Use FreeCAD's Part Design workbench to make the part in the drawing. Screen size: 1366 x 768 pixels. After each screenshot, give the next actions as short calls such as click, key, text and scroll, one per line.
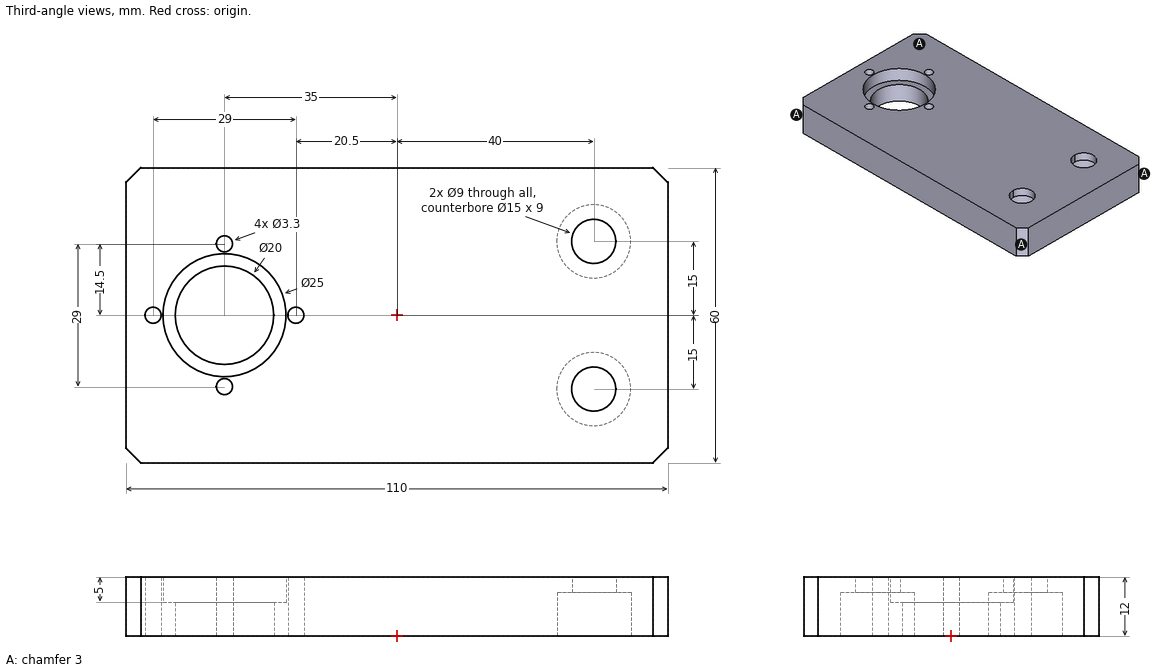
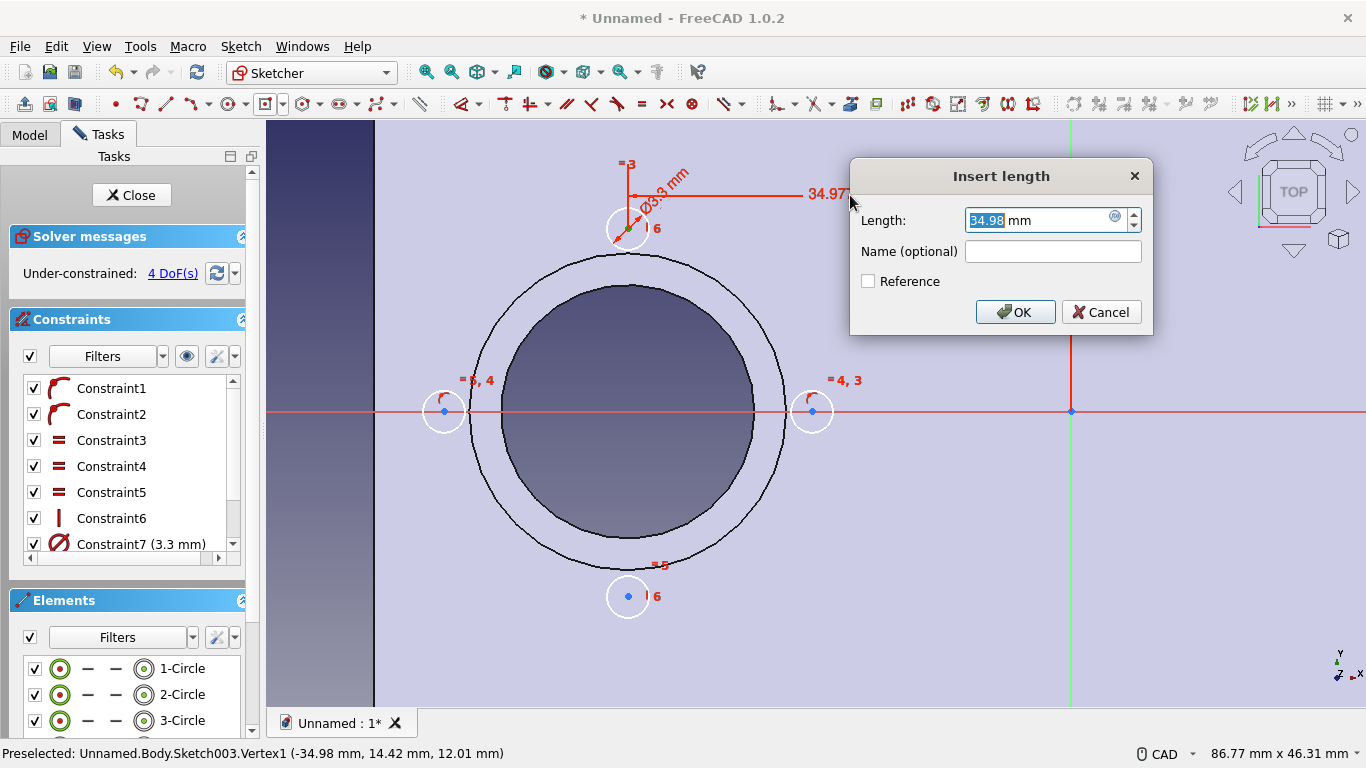
text(35)
key(Return)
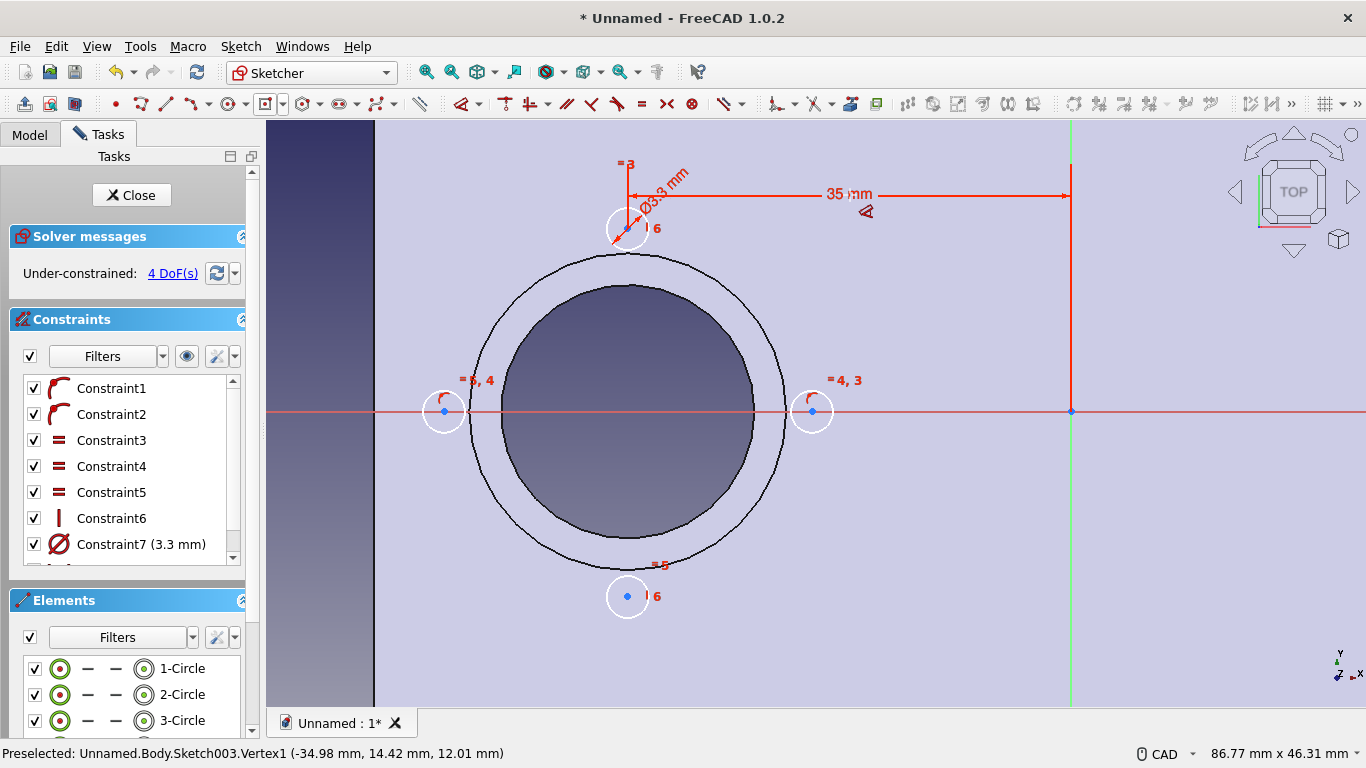
click(812, 412)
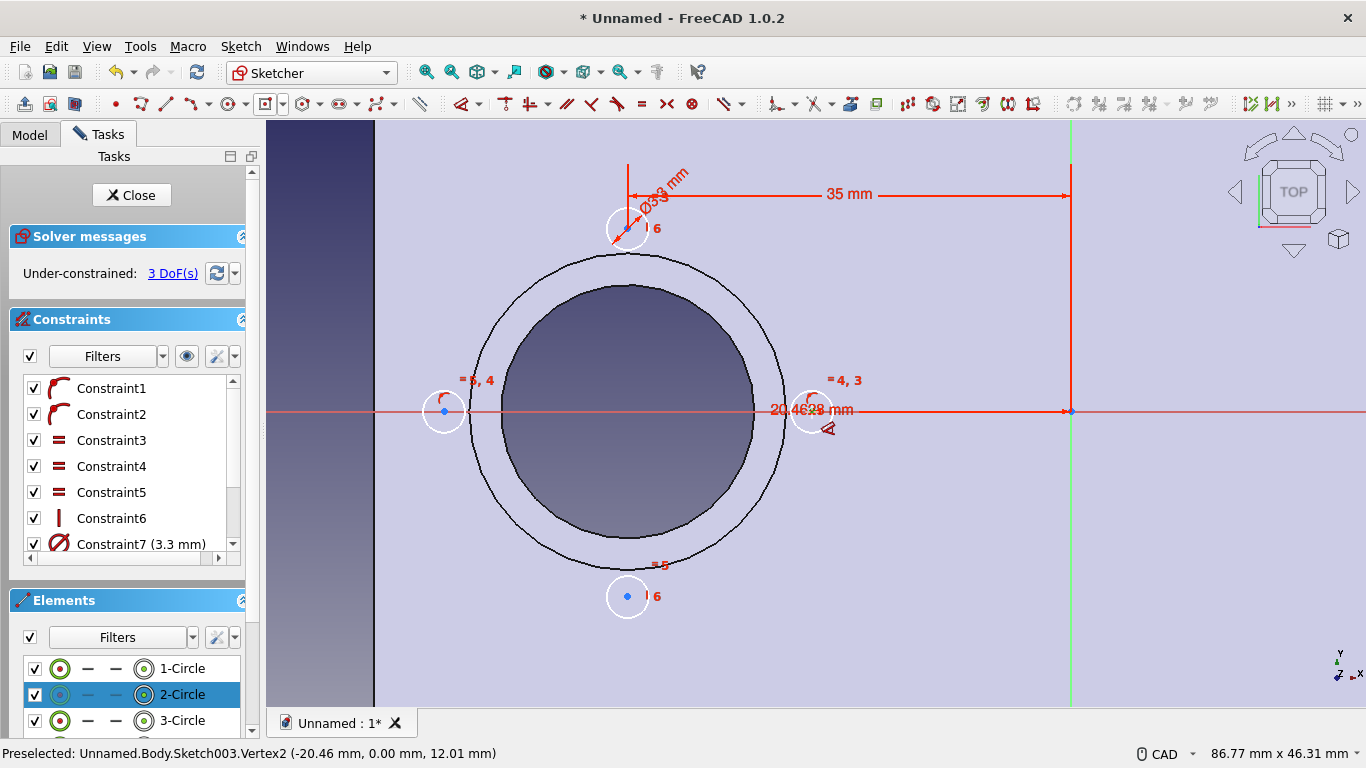
click(444, 412)
click(628, 446)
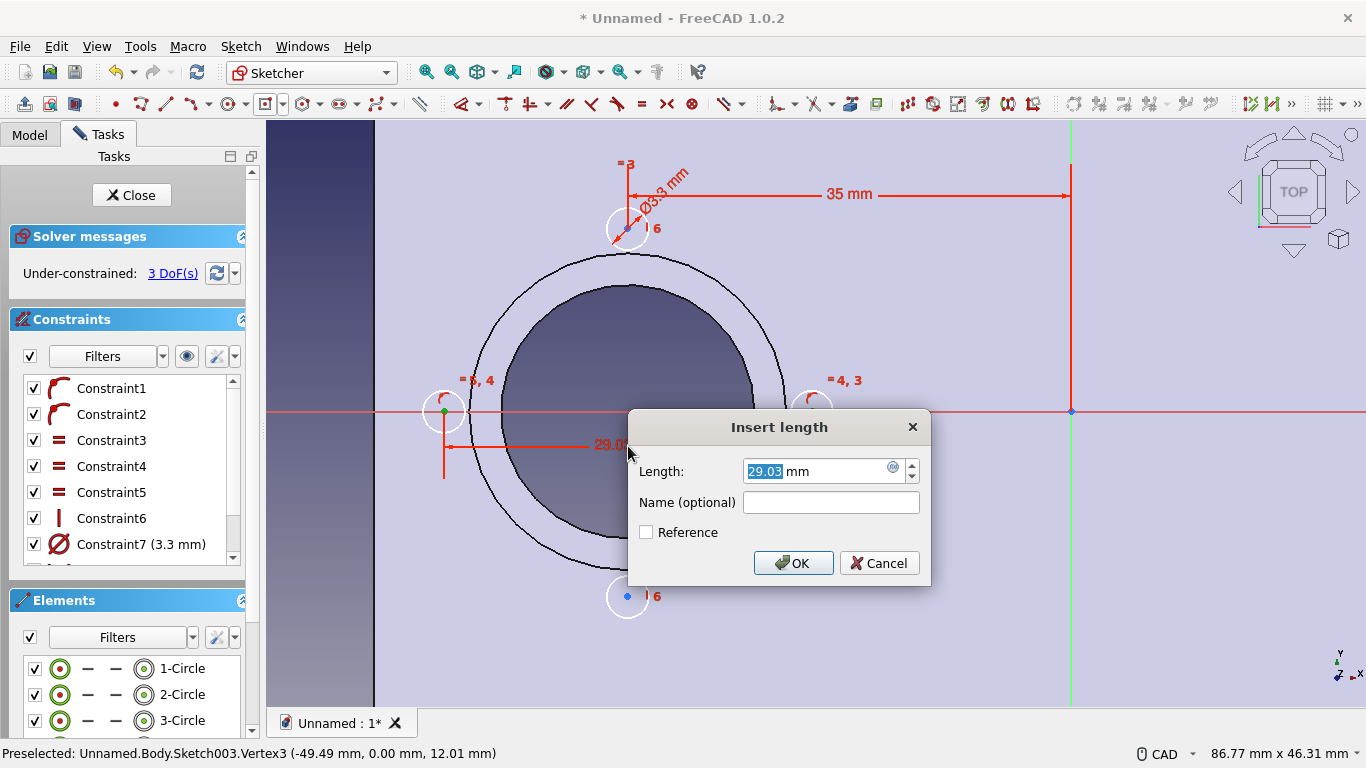
text(29)
key(Return)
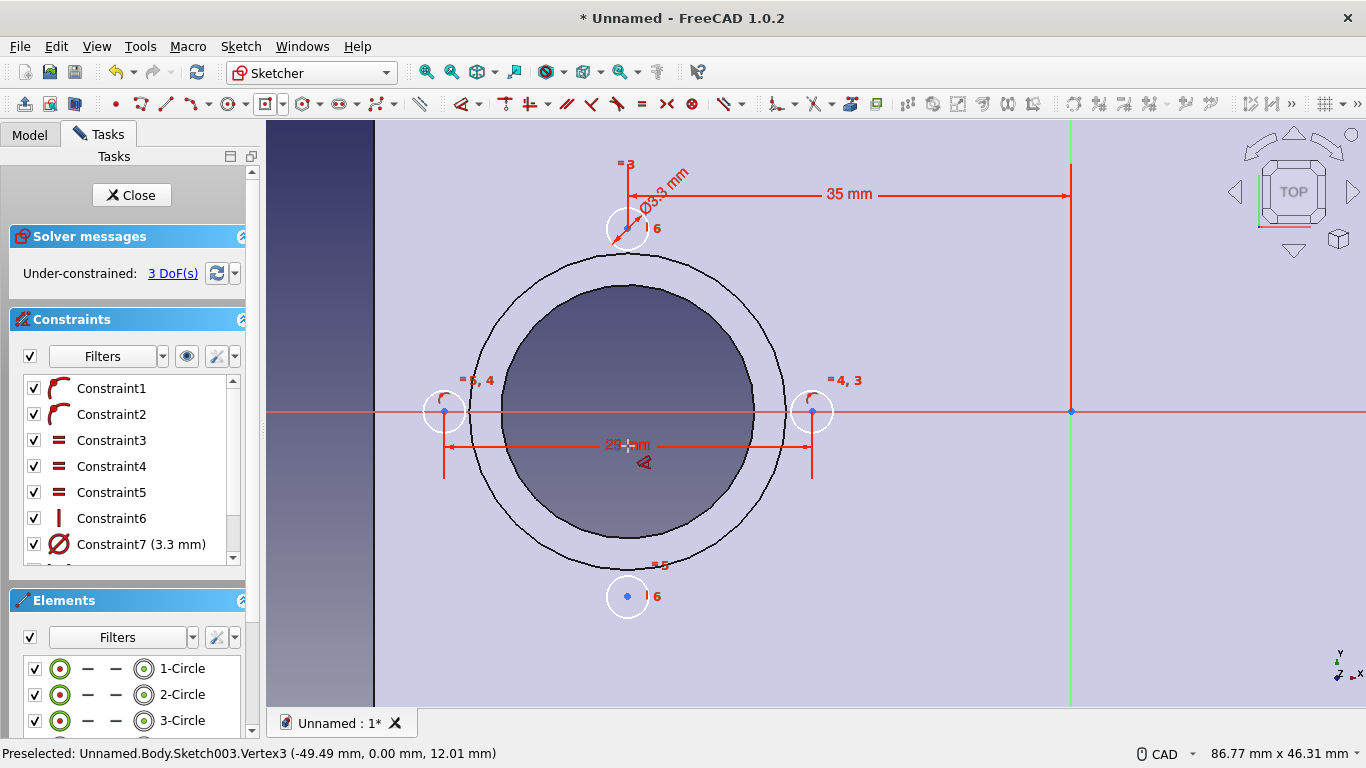
click(628, 229)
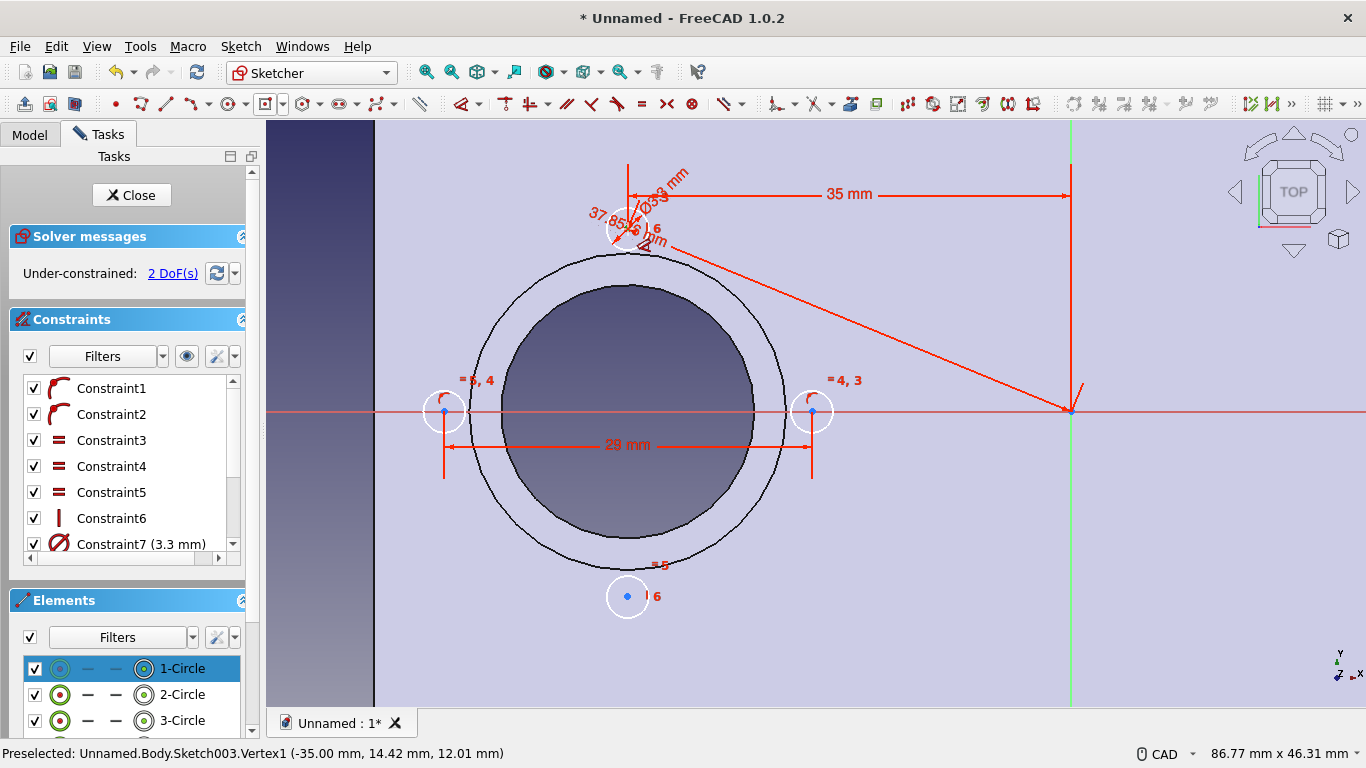
click(628, 597)
click(594, 328)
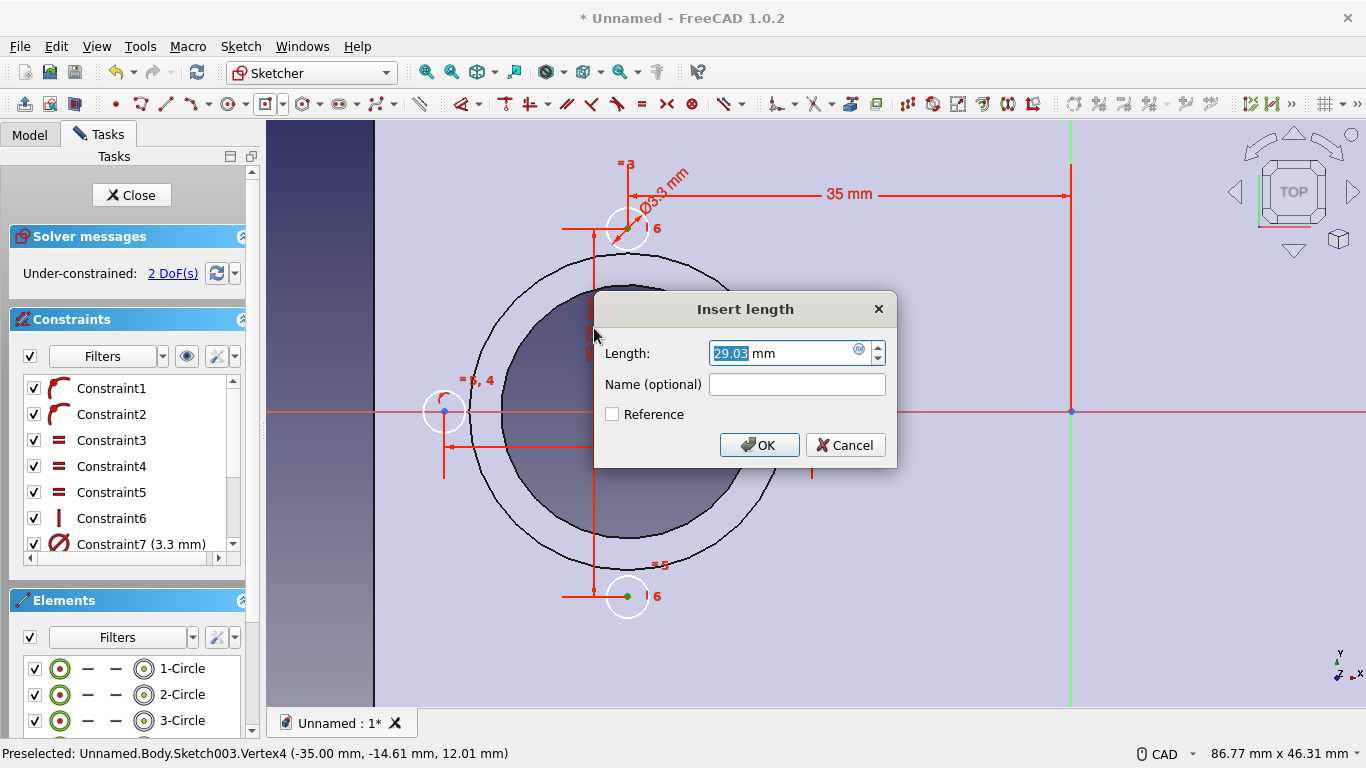
text(29)
key(Return)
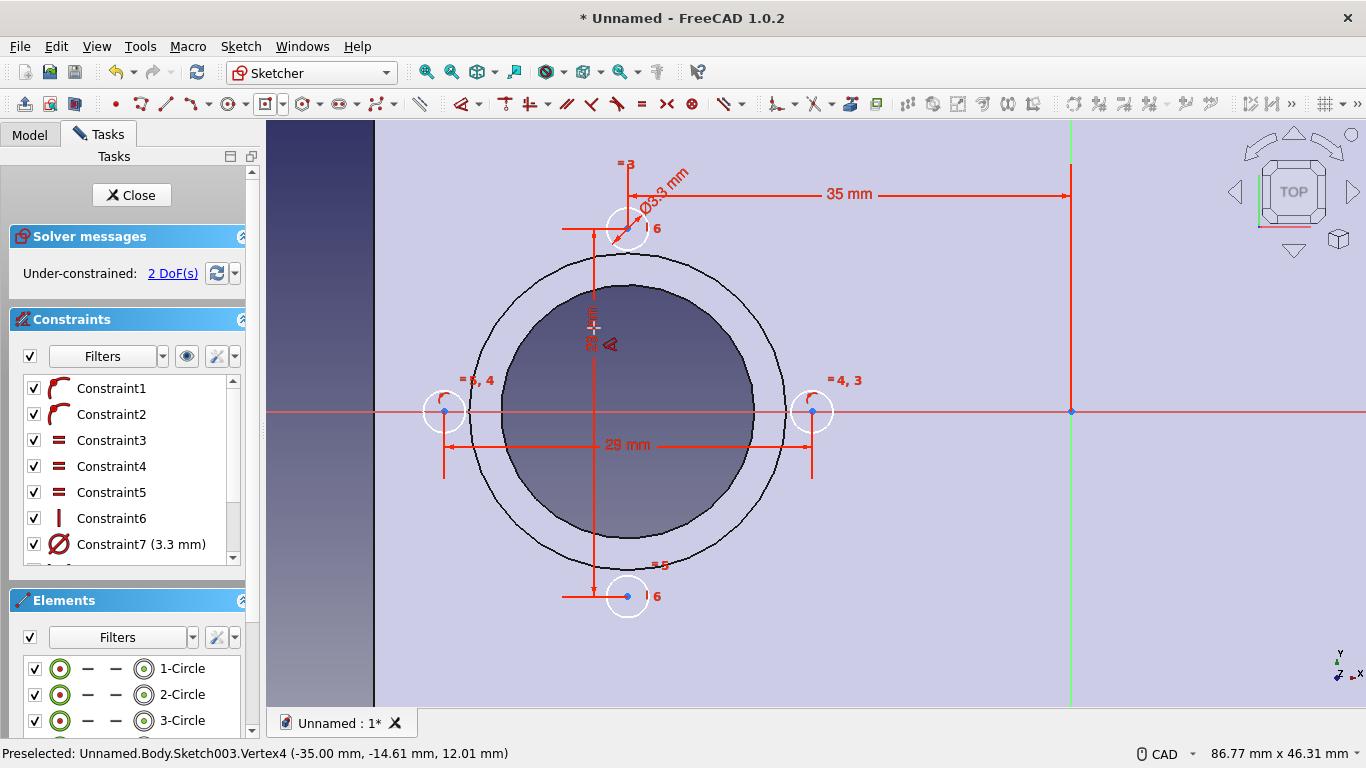
click(628, 229)
click(1105, 320)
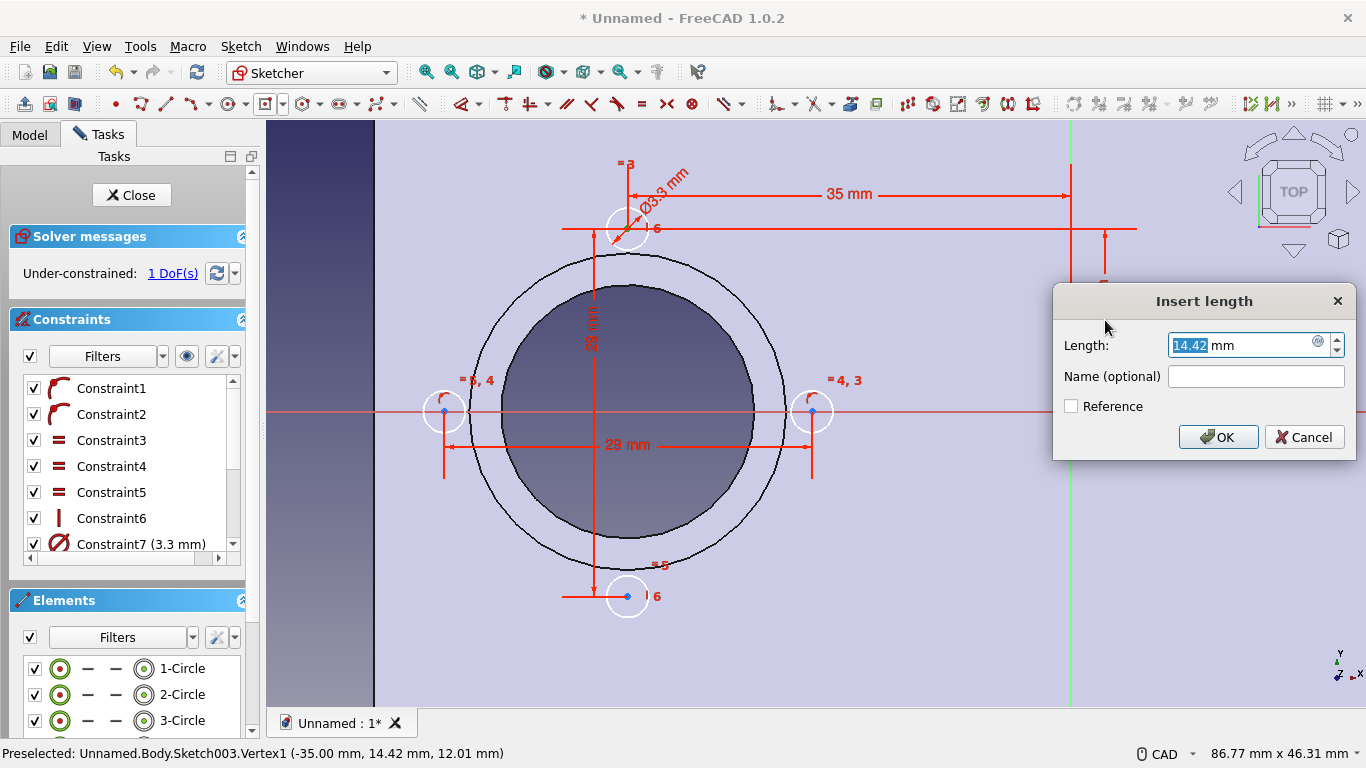
text(14.5)
key(Return)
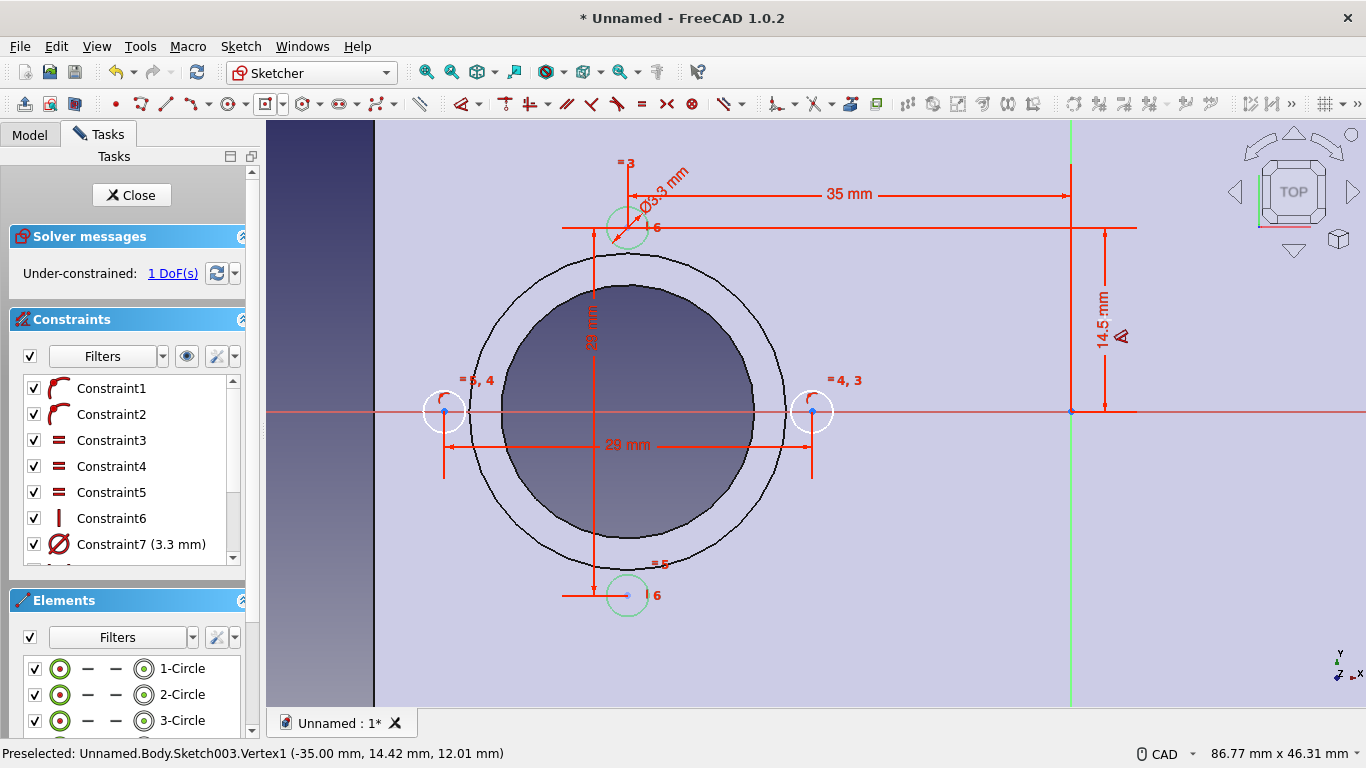
click(812, 412)
click(942, 446)